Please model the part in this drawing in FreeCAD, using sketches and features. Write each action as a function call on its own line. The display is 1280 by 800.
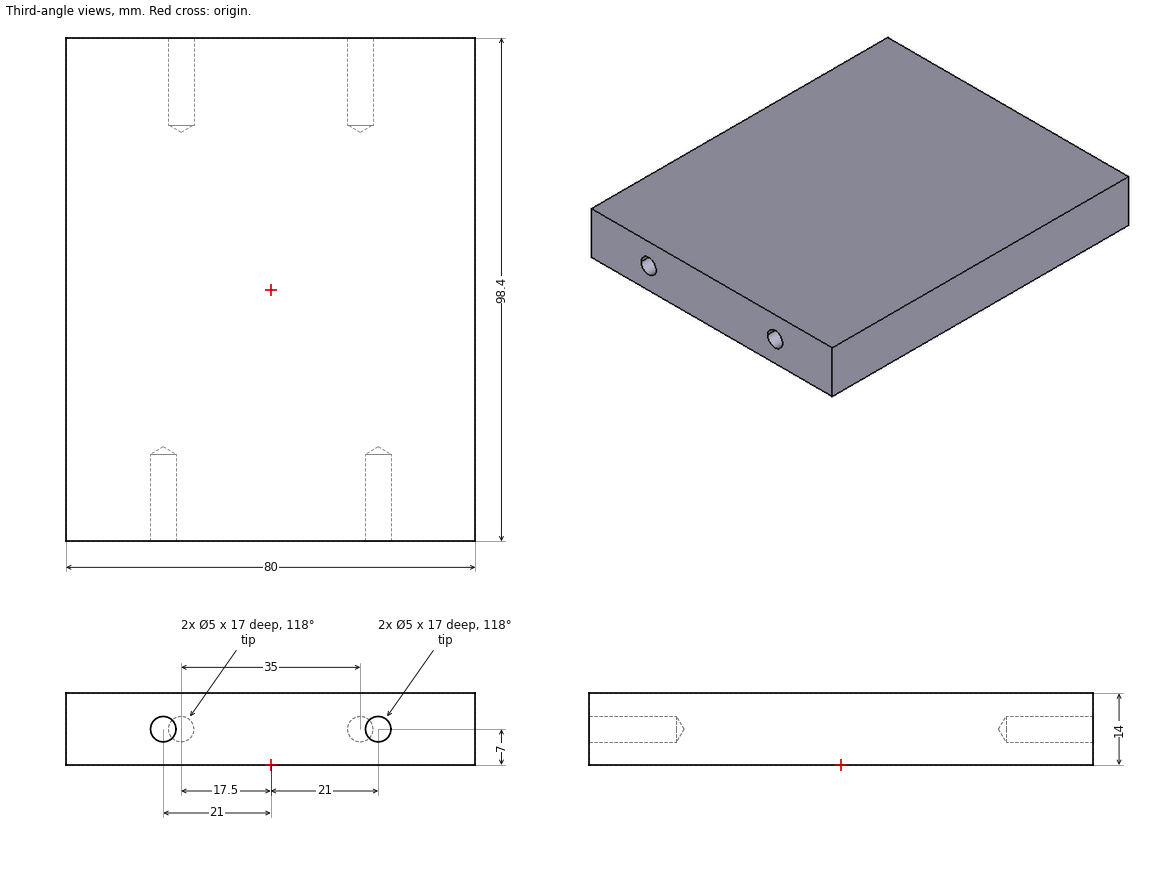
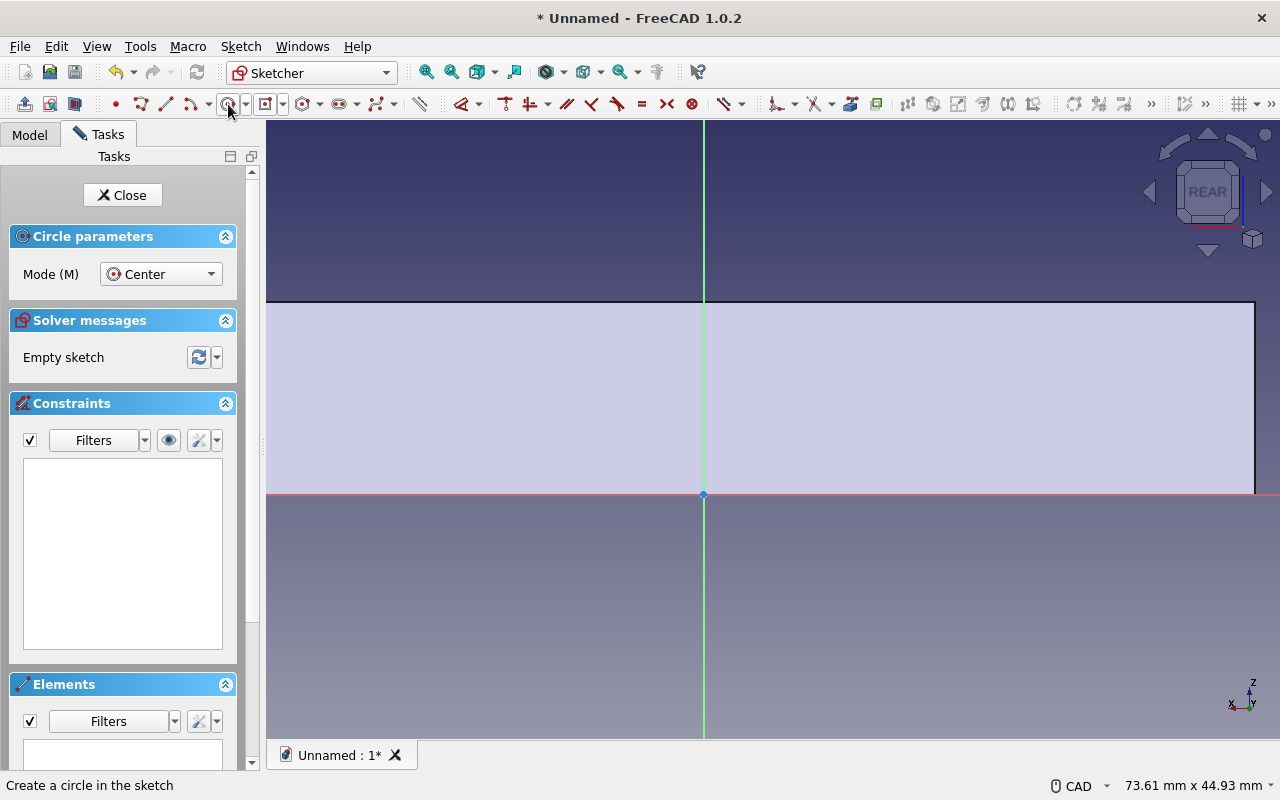
click(945, 398)
click(969, 374)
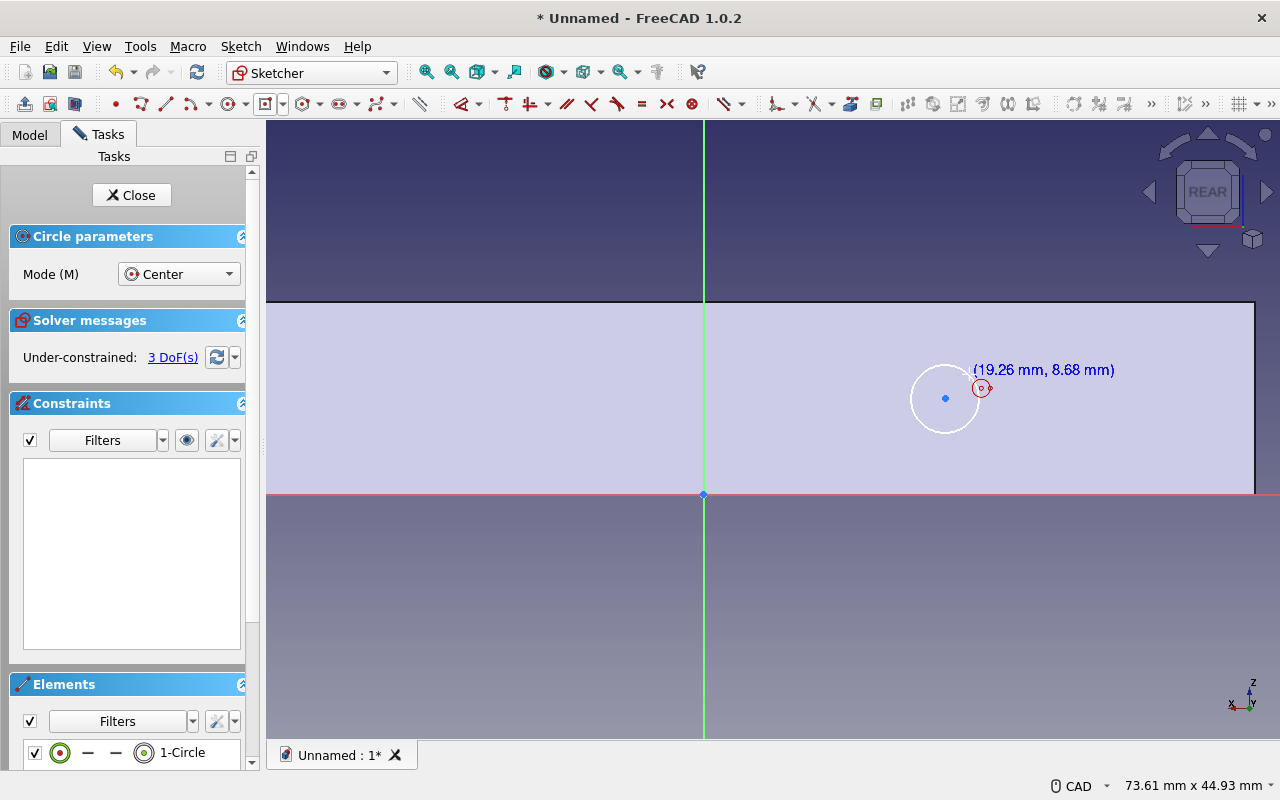
click(463, 398)
click(487, 374)
key(Escape)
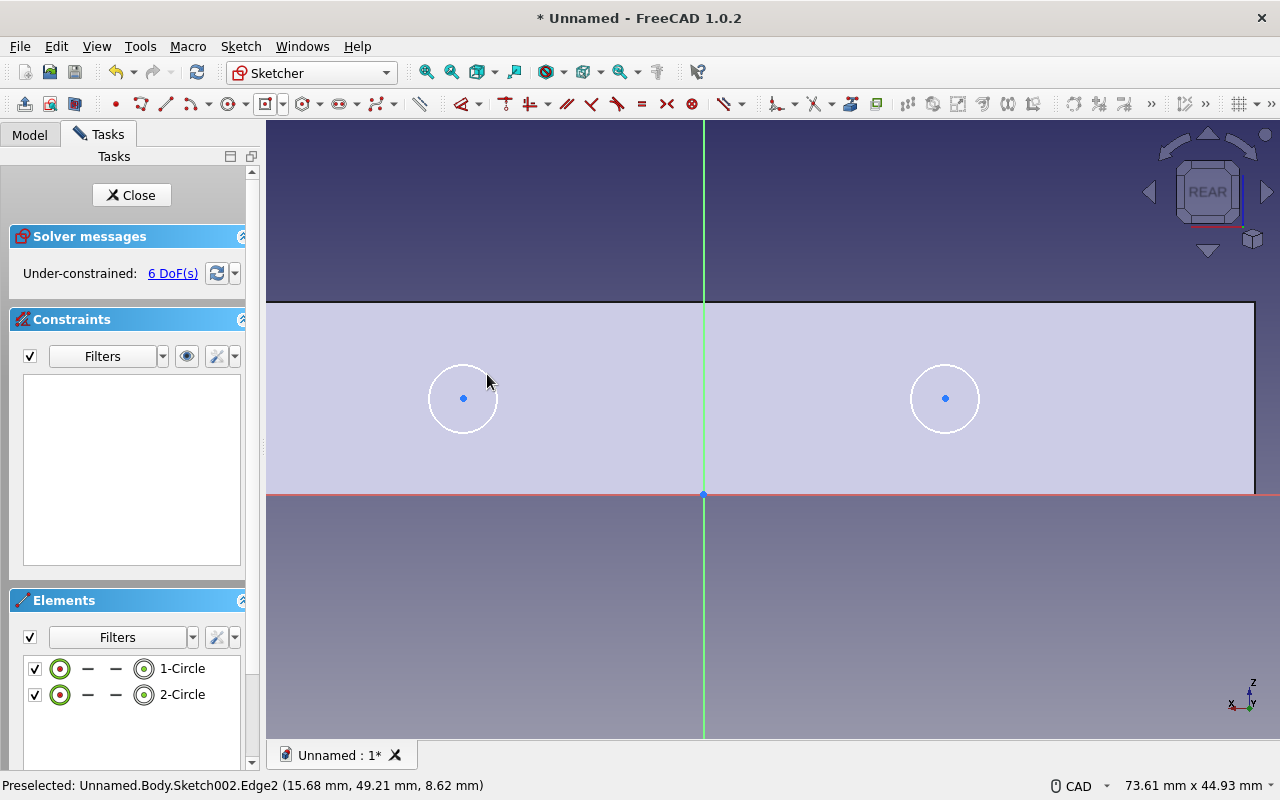
click(969, 375)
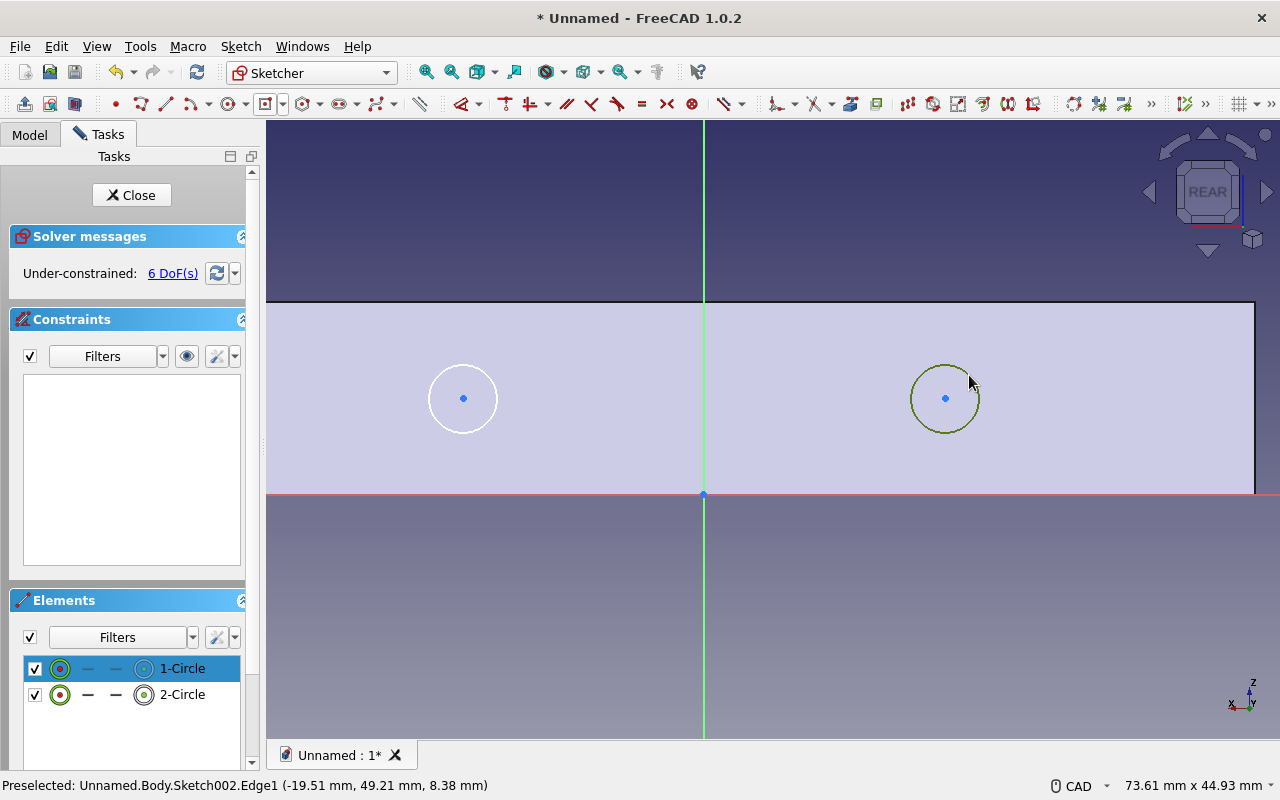
click(487, 375)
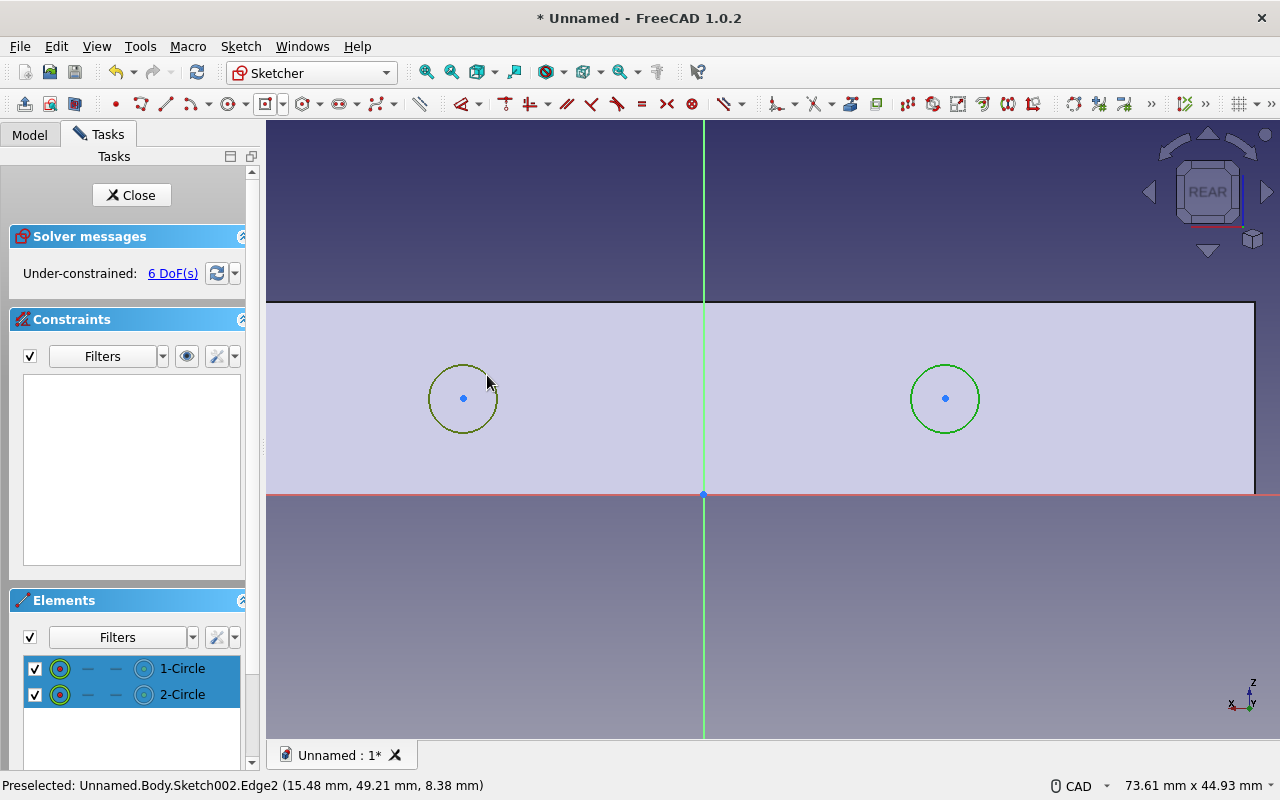
click(642, 104)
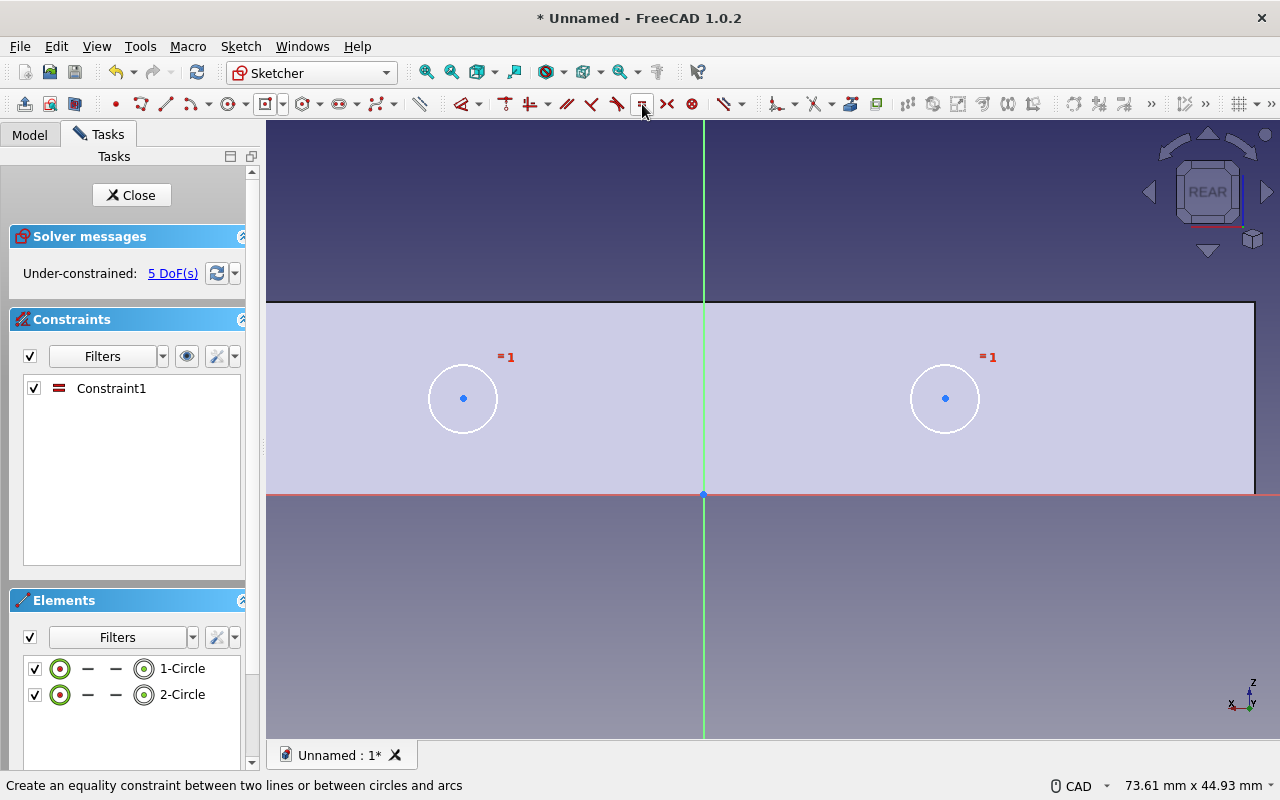
click(945, 399)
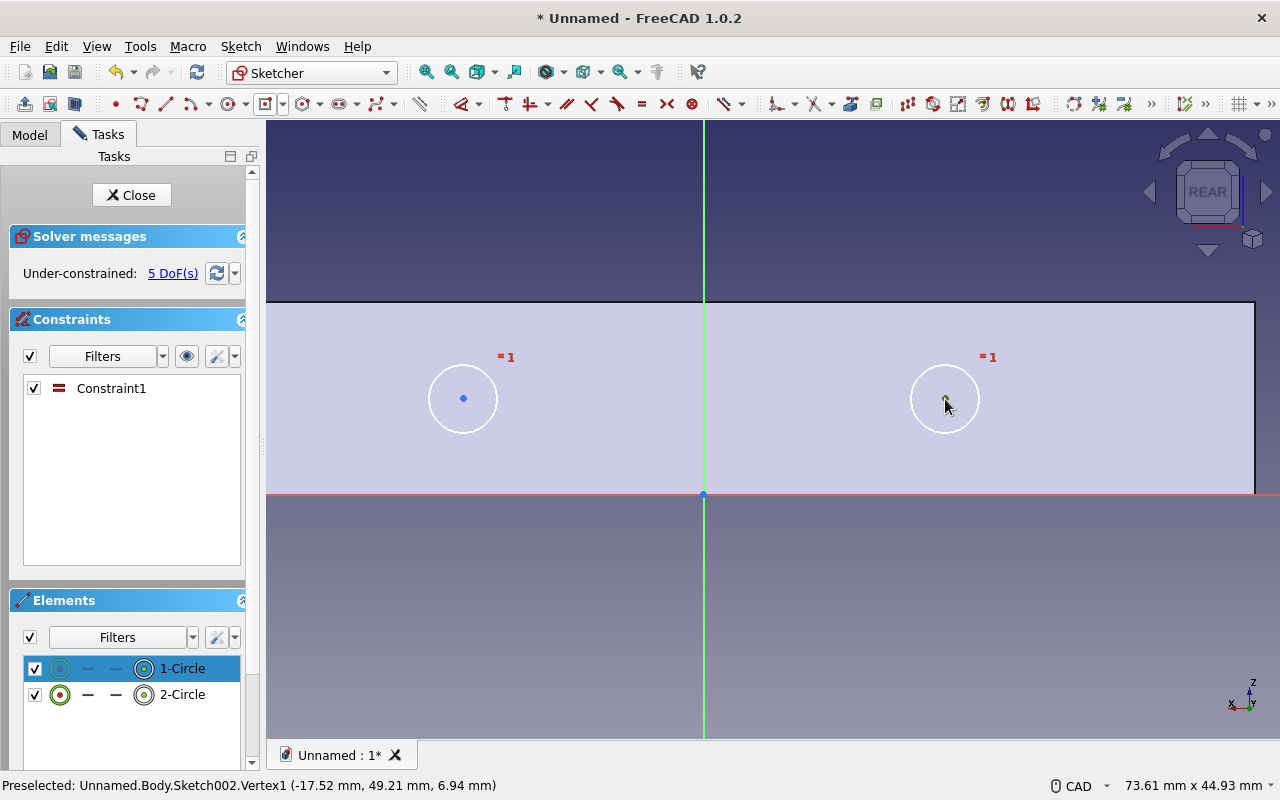
click(463, 399)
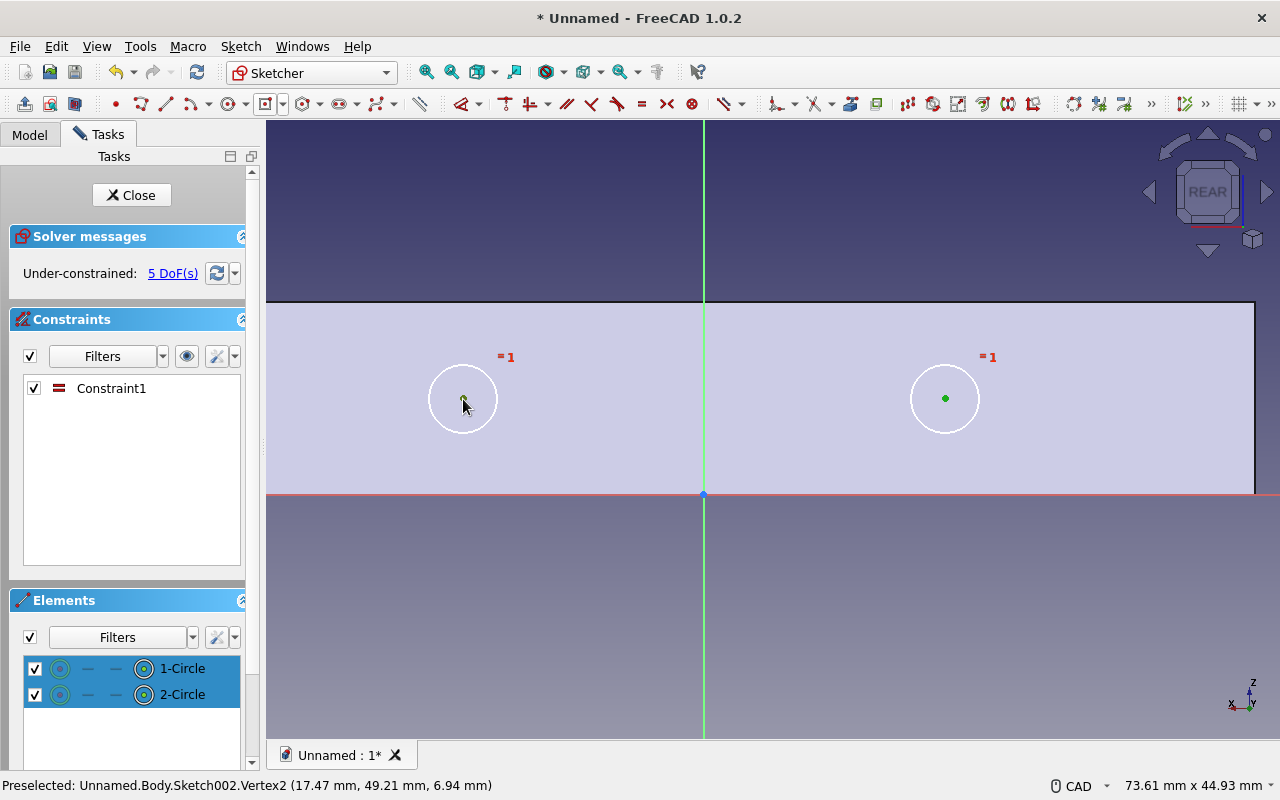
key(h)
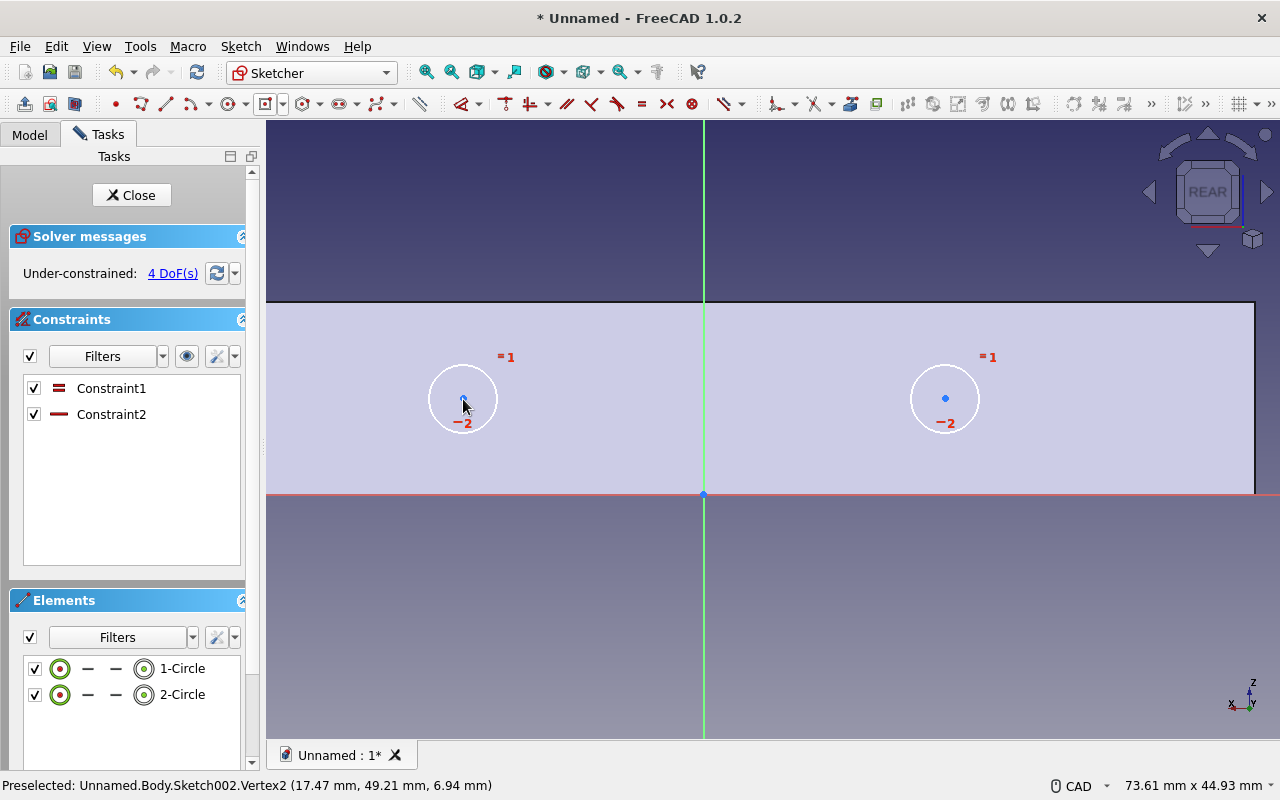
click(460, 104)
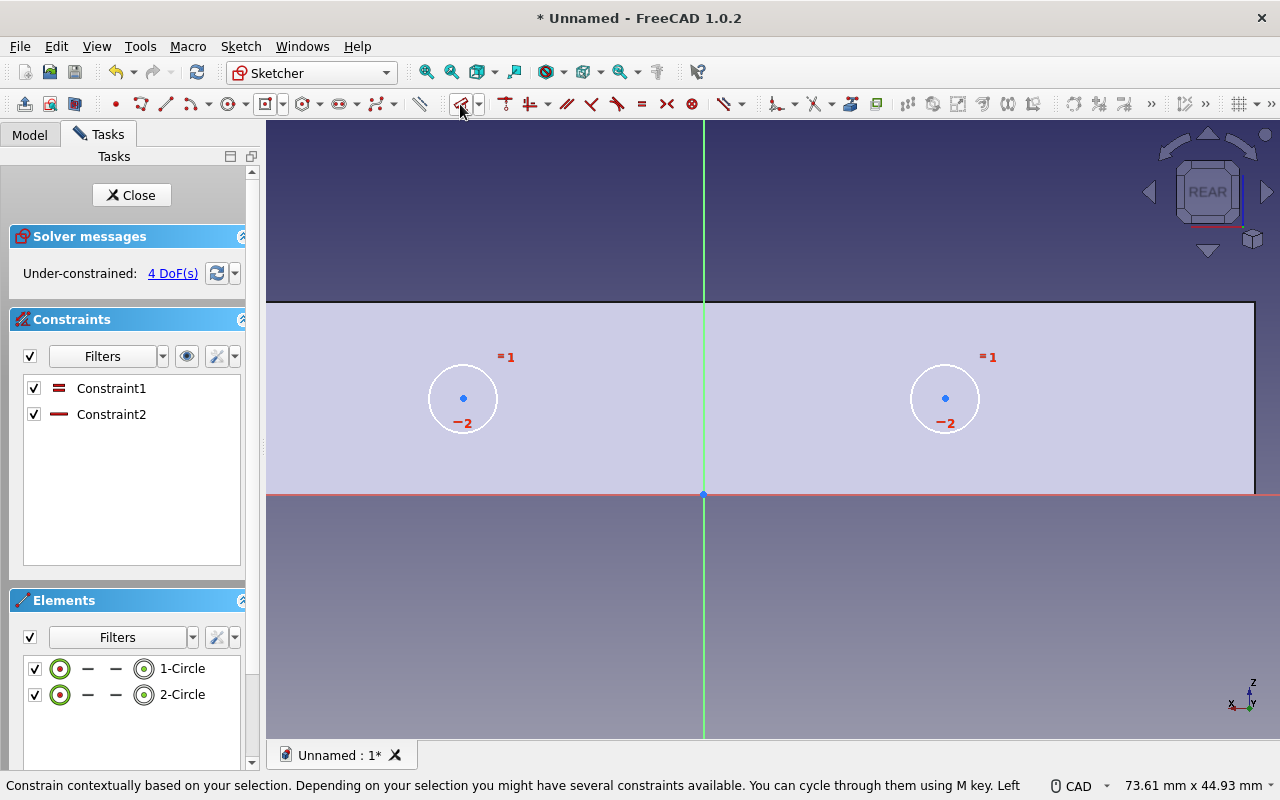
click(969, 375)
click(992, 352)